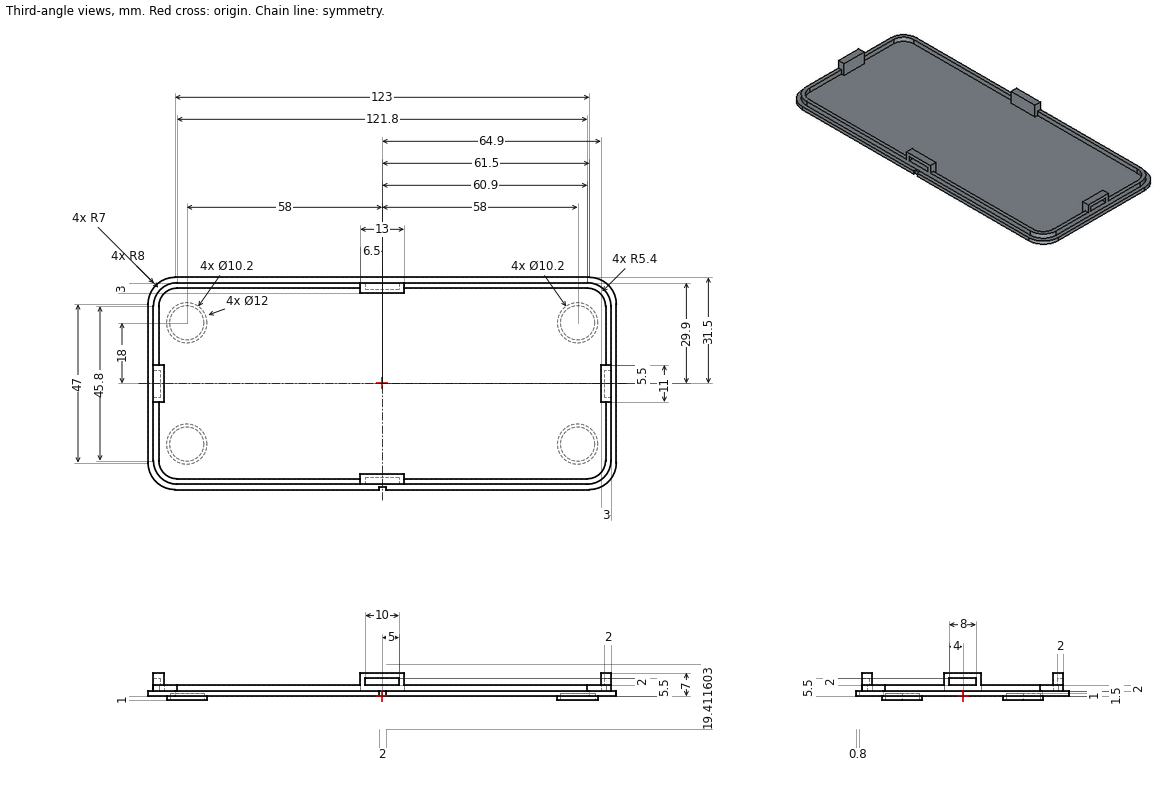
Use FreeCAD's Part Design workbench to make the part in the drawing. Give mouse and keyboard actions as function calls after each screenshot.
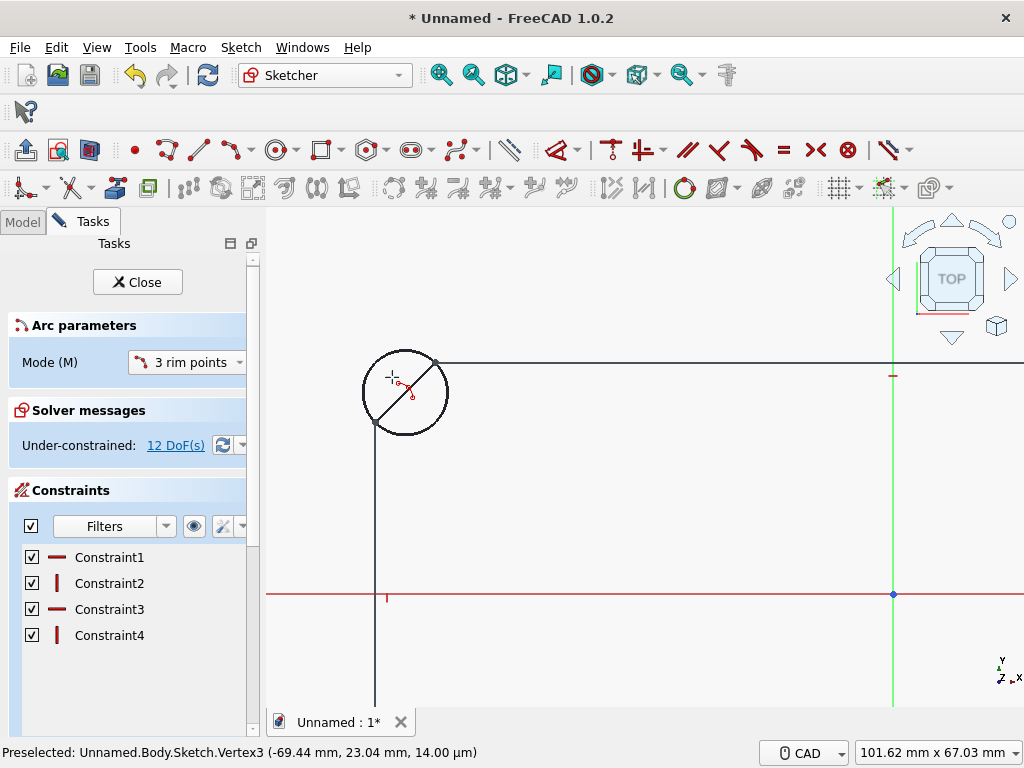
click(392, 377)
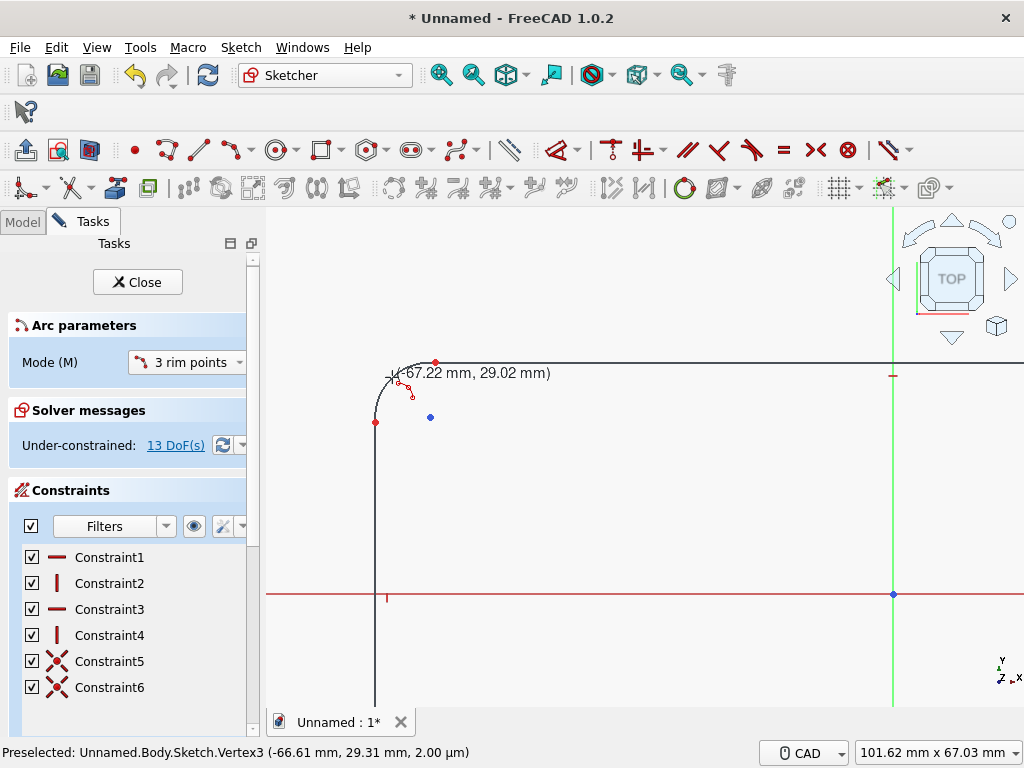
scroll(392, 377, down, 5)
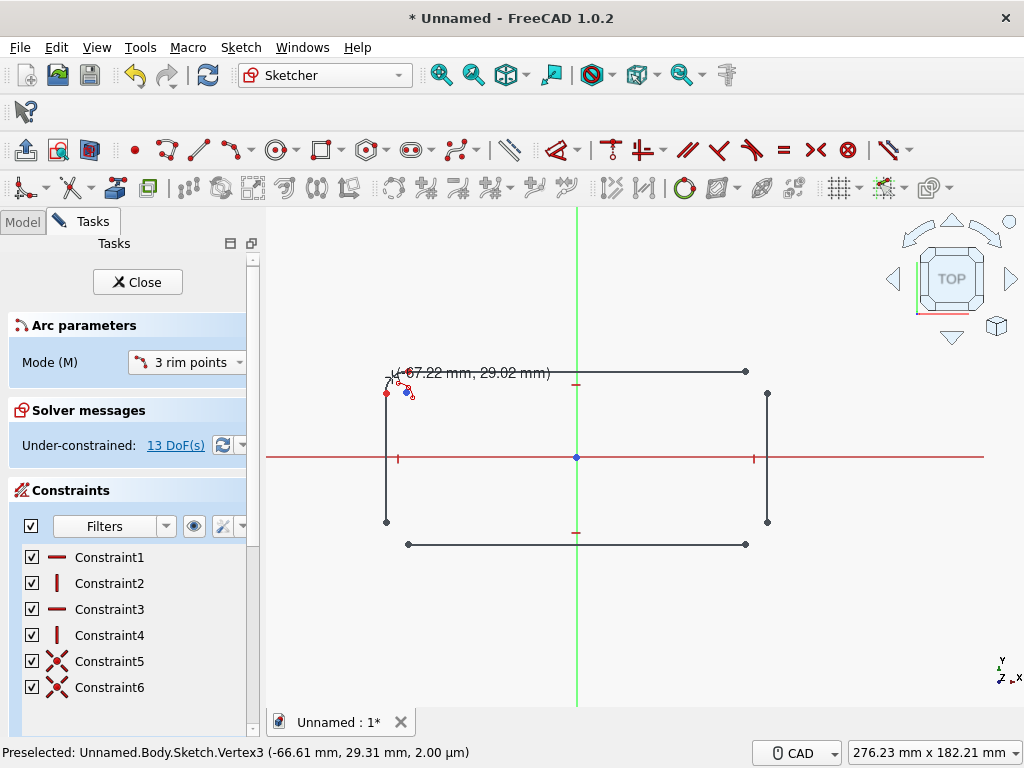
click(386, 523)
click(408, 545)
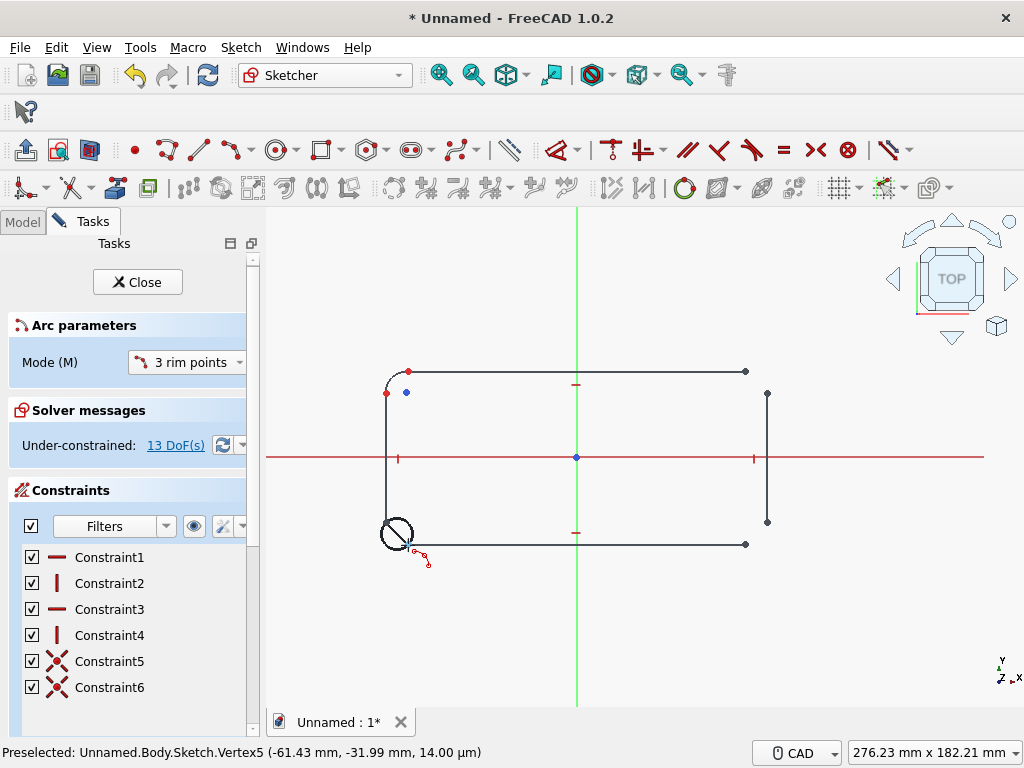
scroll(392, 537, up, 5)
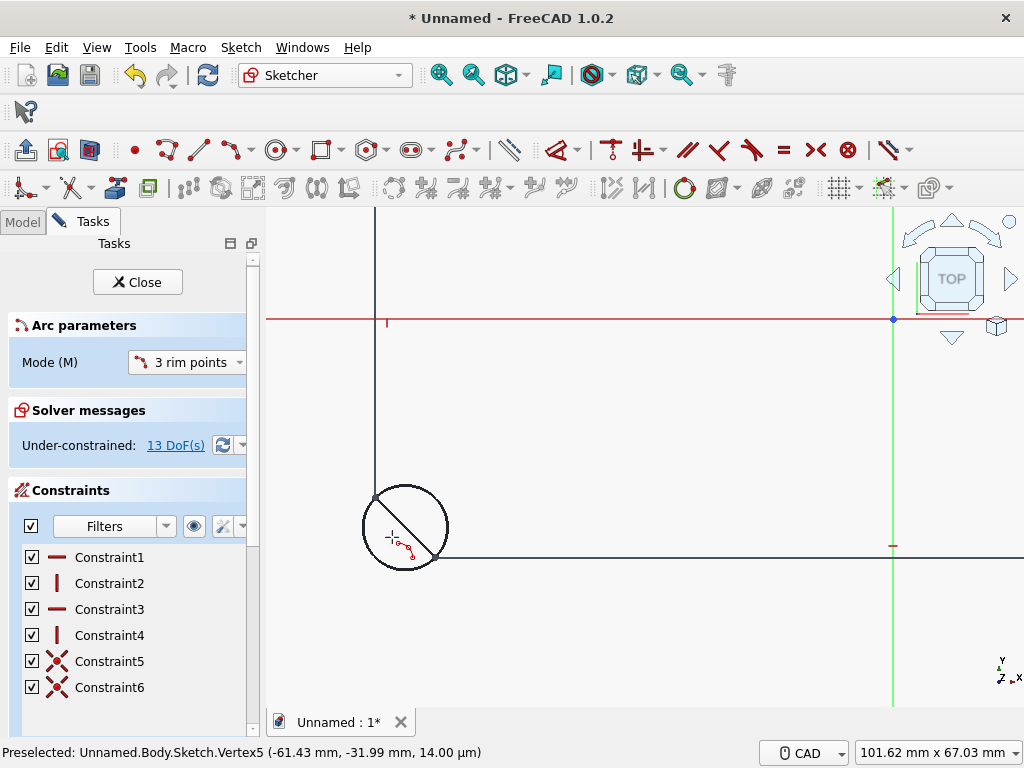
click(392, 537)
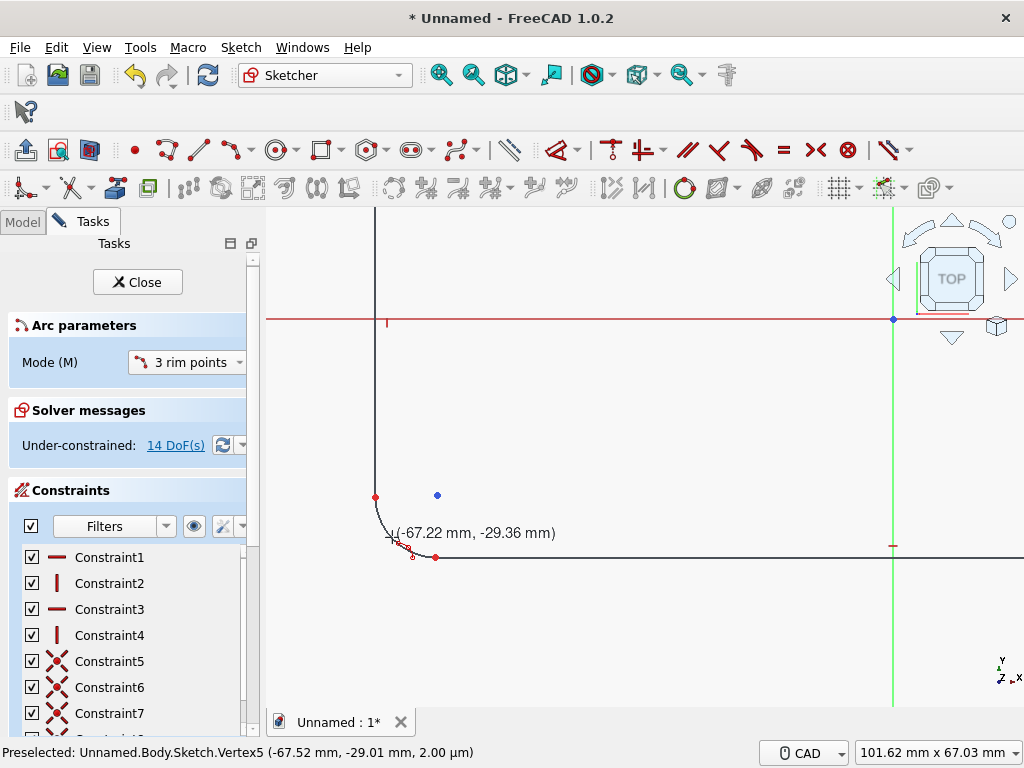
scroll(392, 537, down, 5)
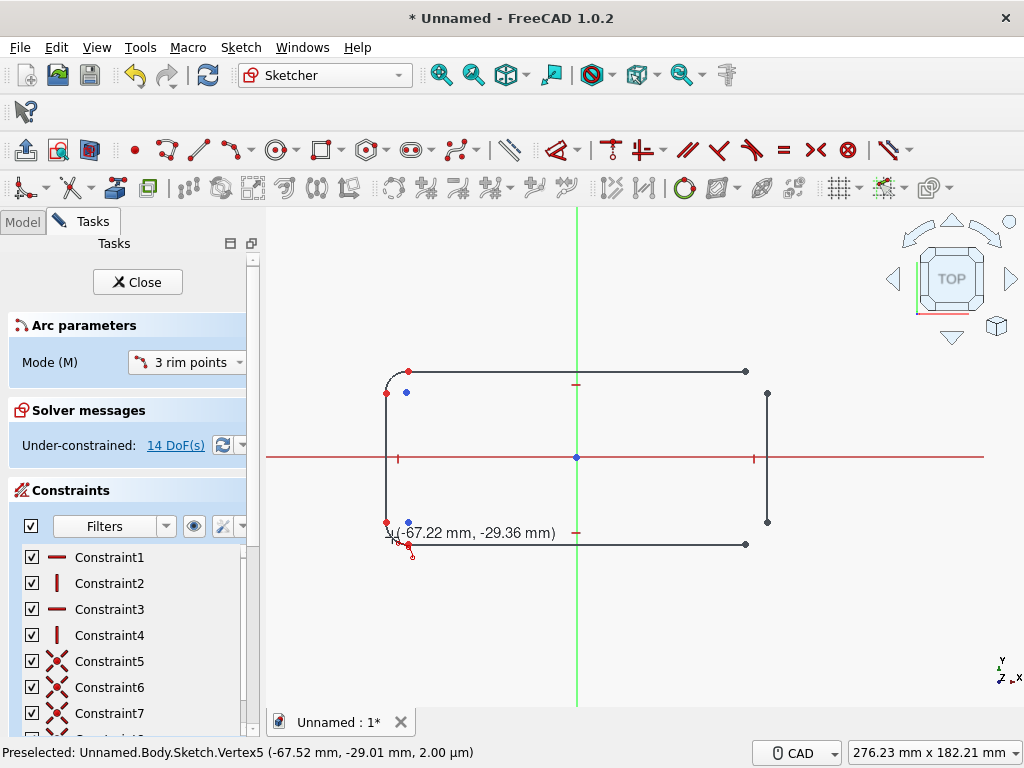
click(745, 545)
click(767, 523)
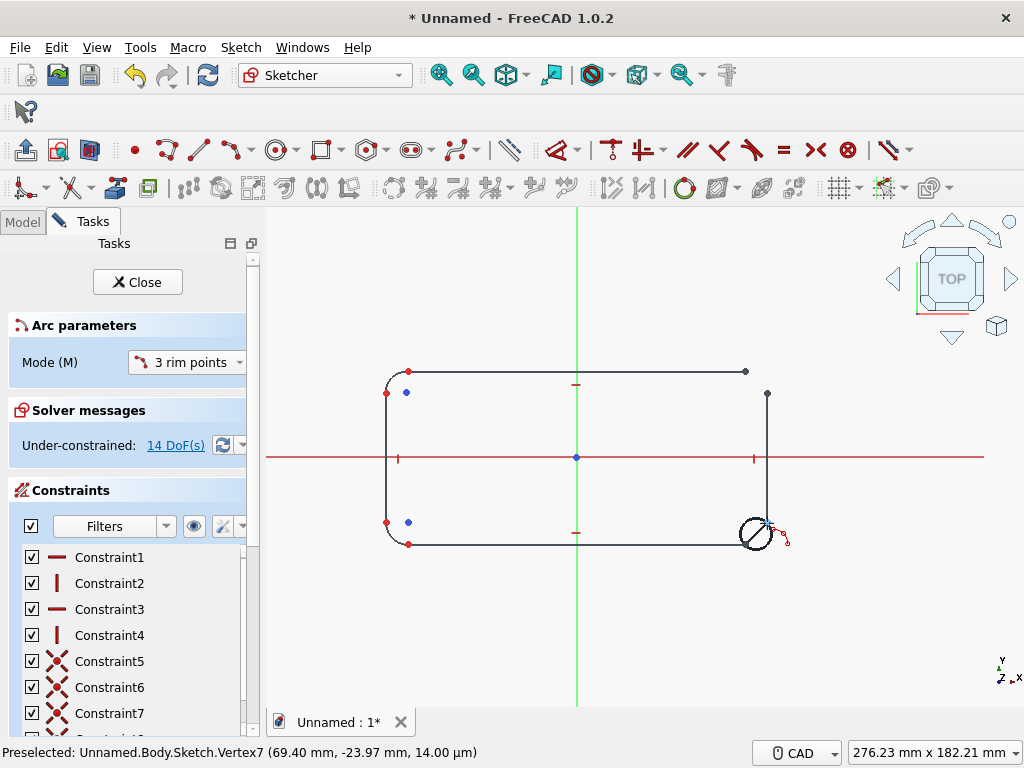
scroll(761, 537, up, 5)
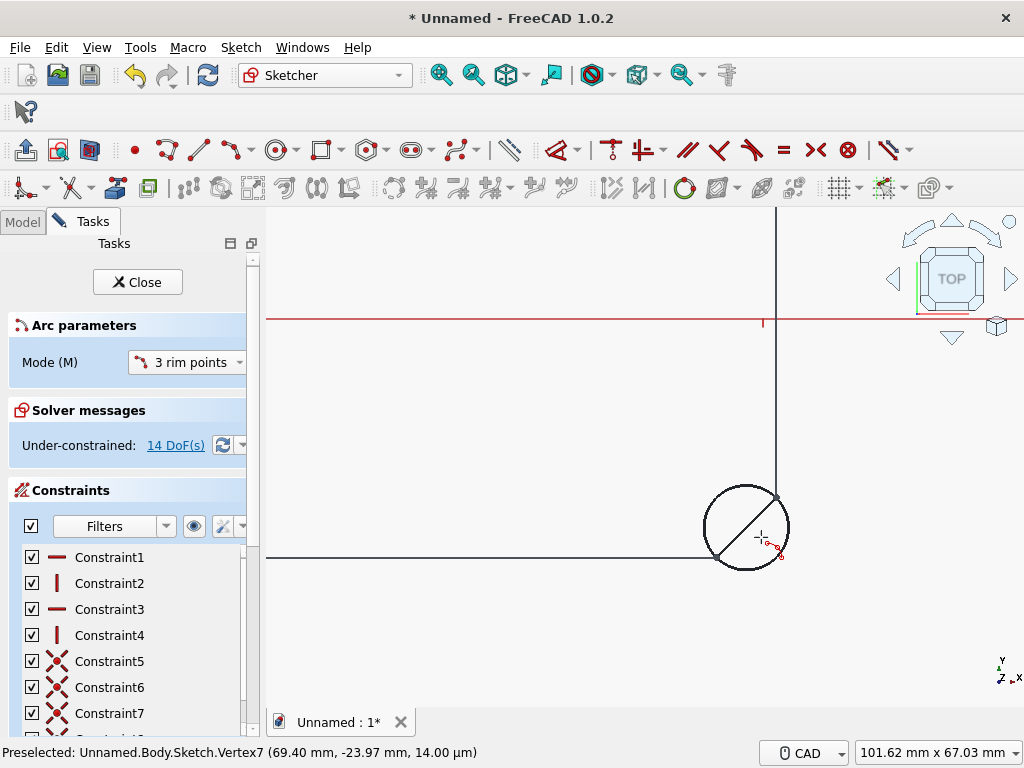
click(759, 537)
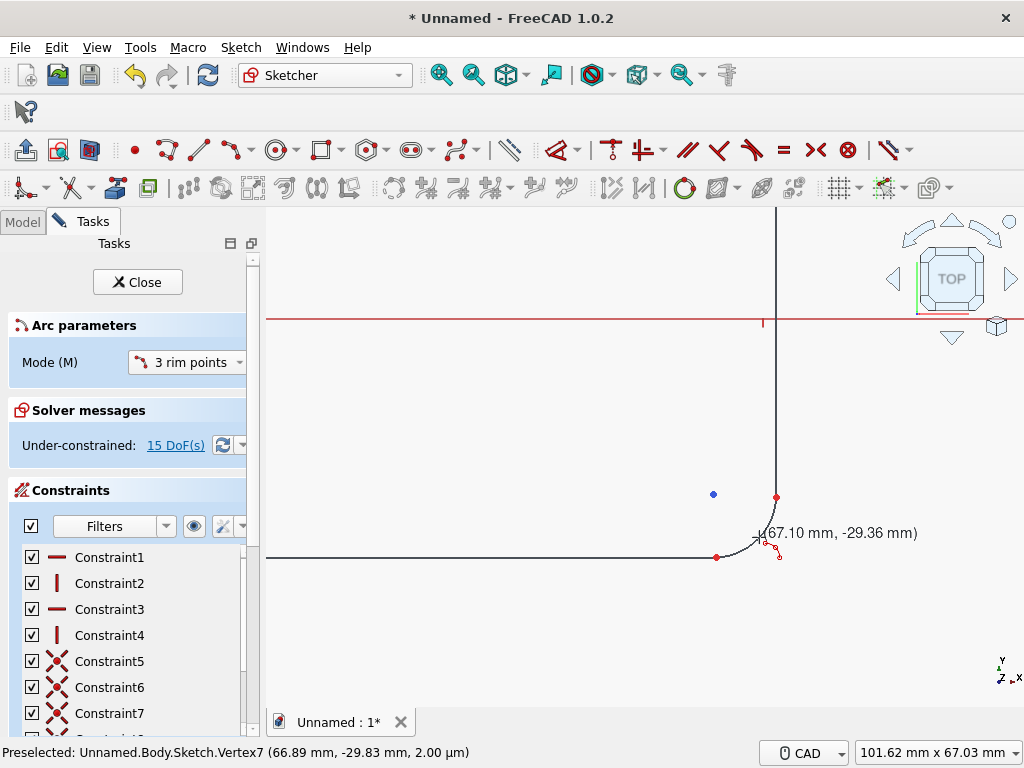
scroll(762, 537, down, 5)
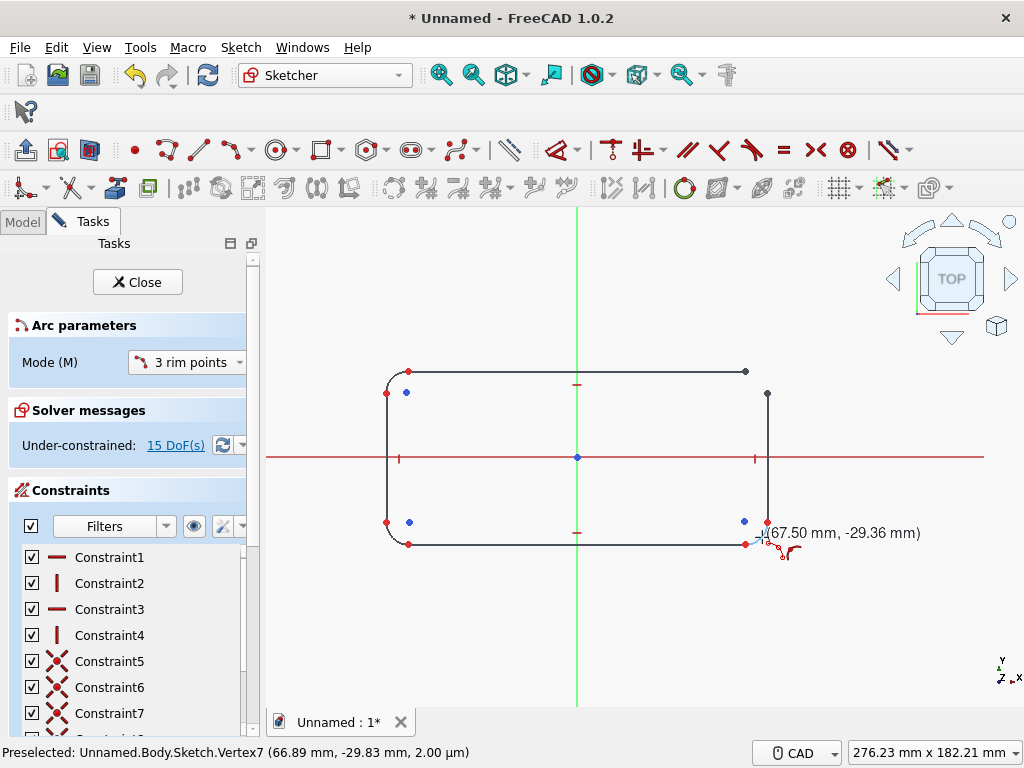
click(768, 394)
click(746, 372)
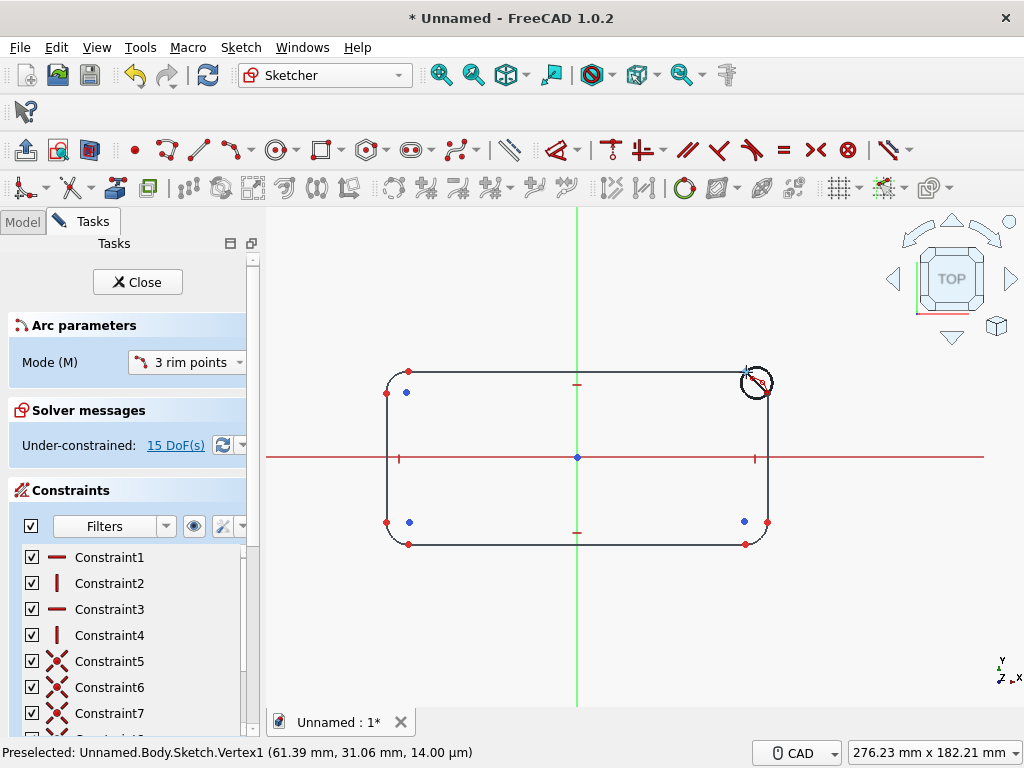
scroll(761, 377, up, 5)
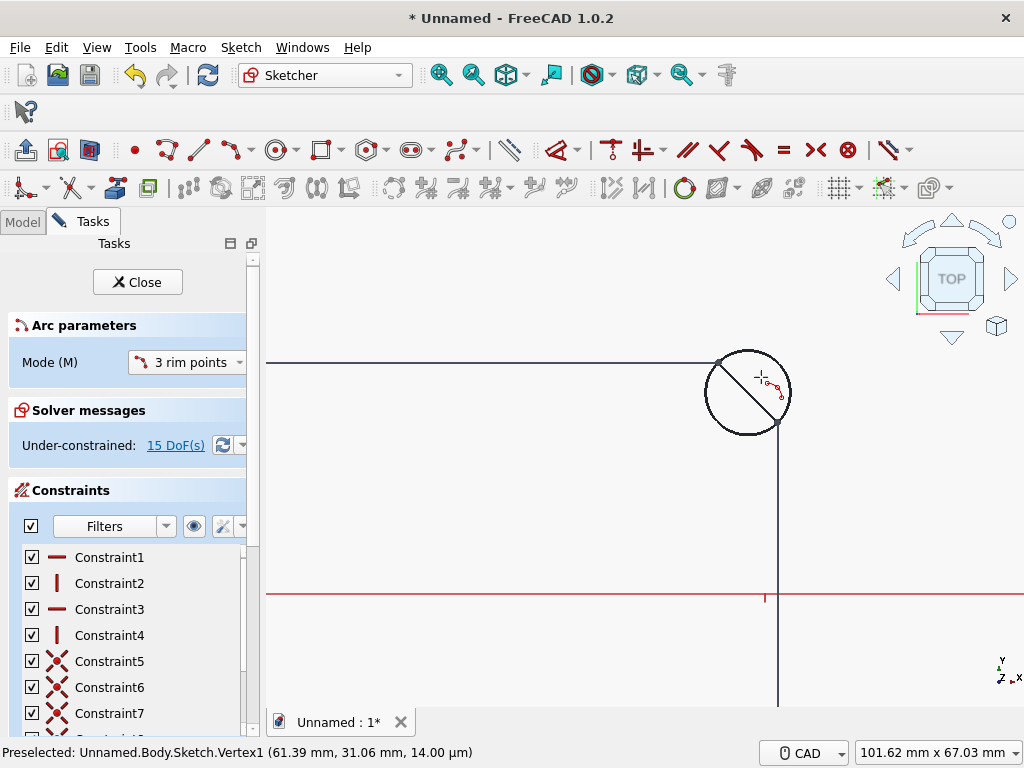
click(761, 377)
key(Escape)